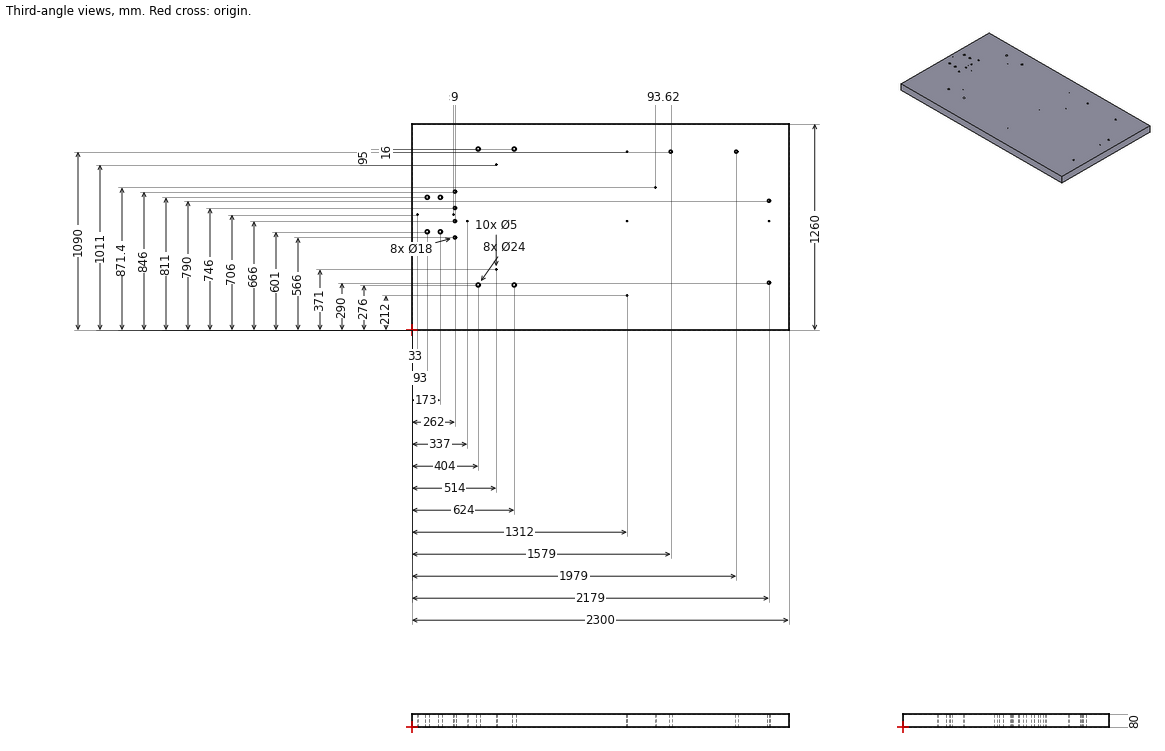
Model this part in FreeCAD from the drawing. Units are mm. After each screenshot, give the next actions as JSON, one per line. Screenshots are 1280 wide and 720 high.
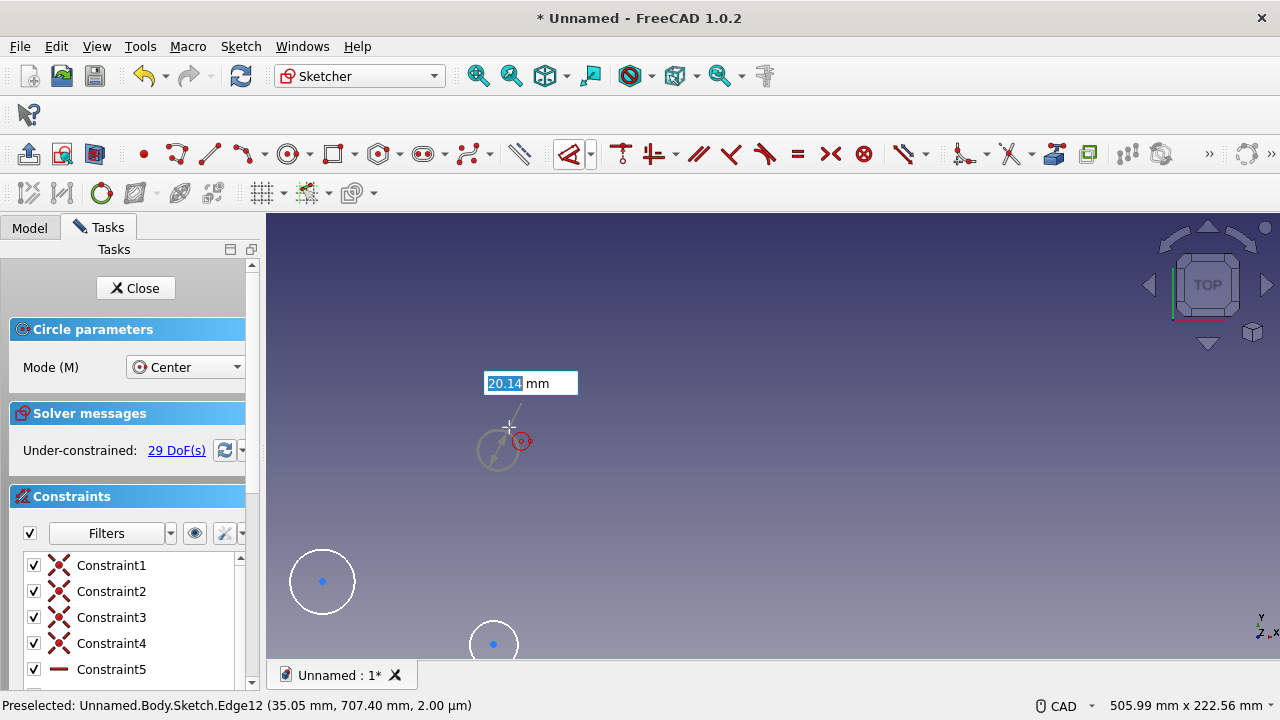
{"action": "left_click", "coordinate": [510, 425]}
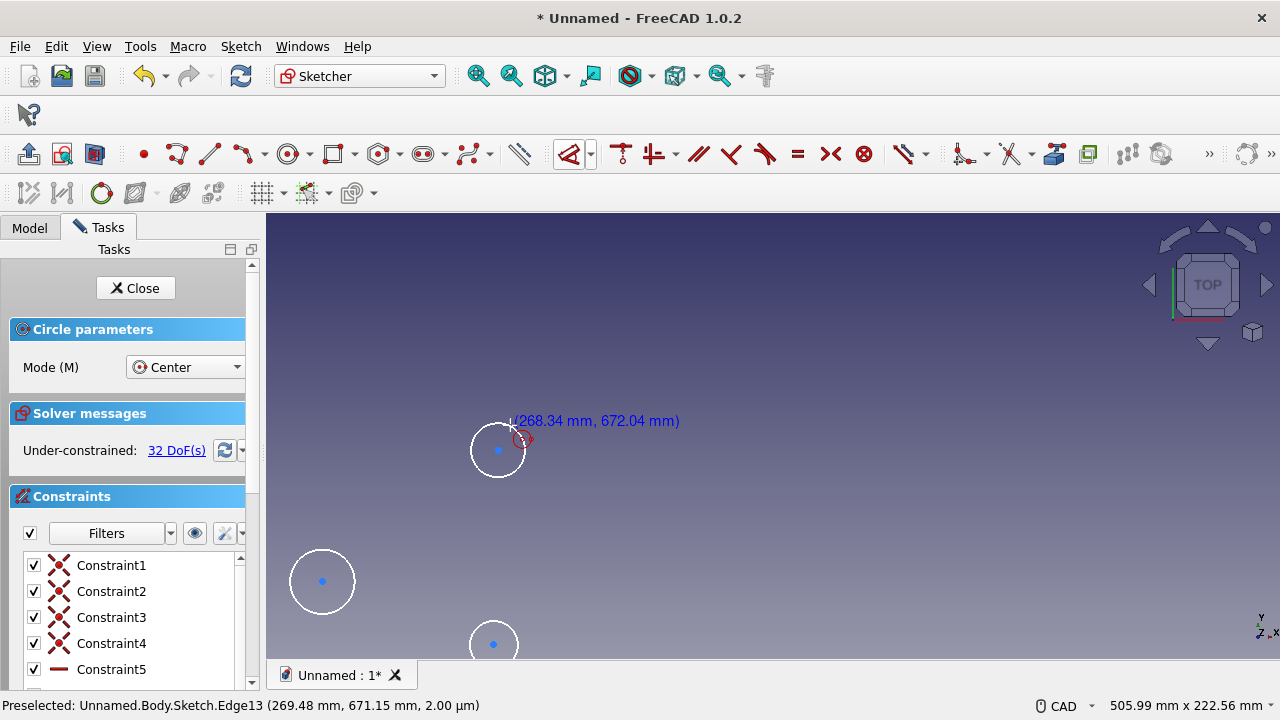
{"action": "scroll", "coordinate": [479, 358], "scroll_direction": "up", "scroll_amount": 8}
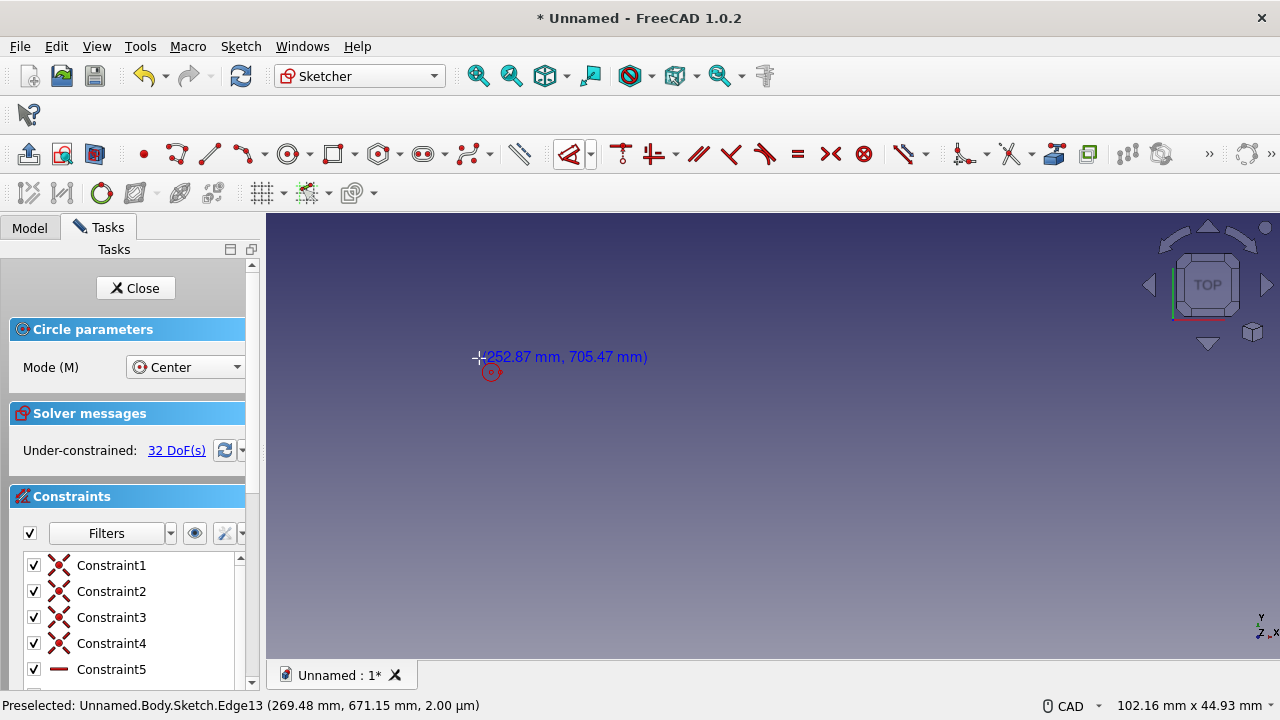
{"action": "scroll", "coordinate": [704, 436], "scroll_direction": "down", "scroll_amount": 15}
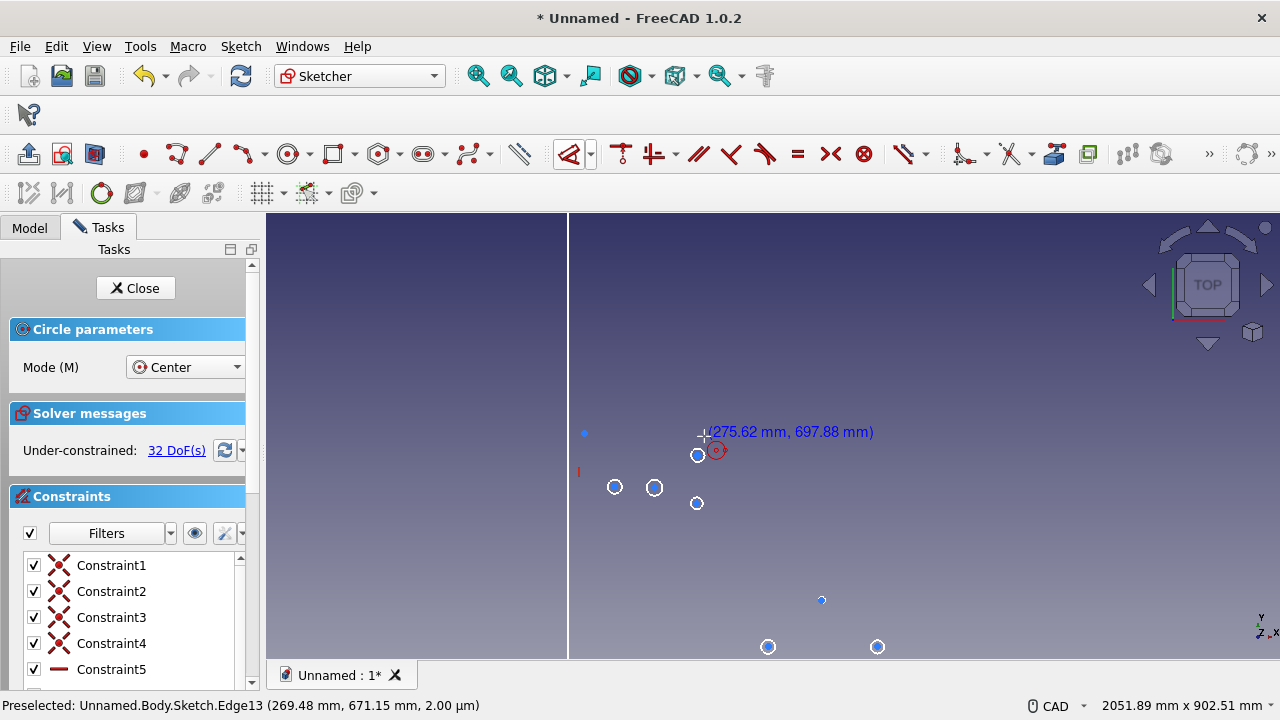
{"action": "scroll", "coordinate": [352, 408], "scroll_direction": "down", "scroll_amount": 4}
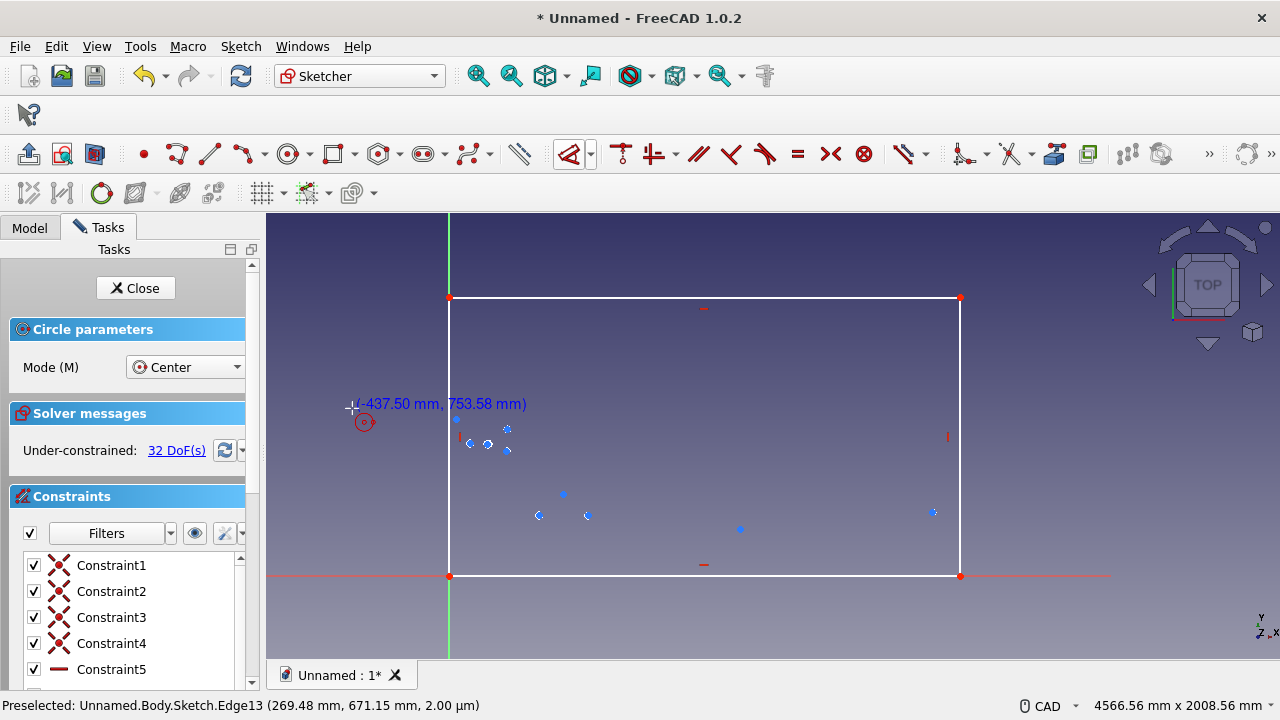
{"action": "scroll", "coordinate": [505, 419], "scroll_direction": "up", "scroll_amount": 5}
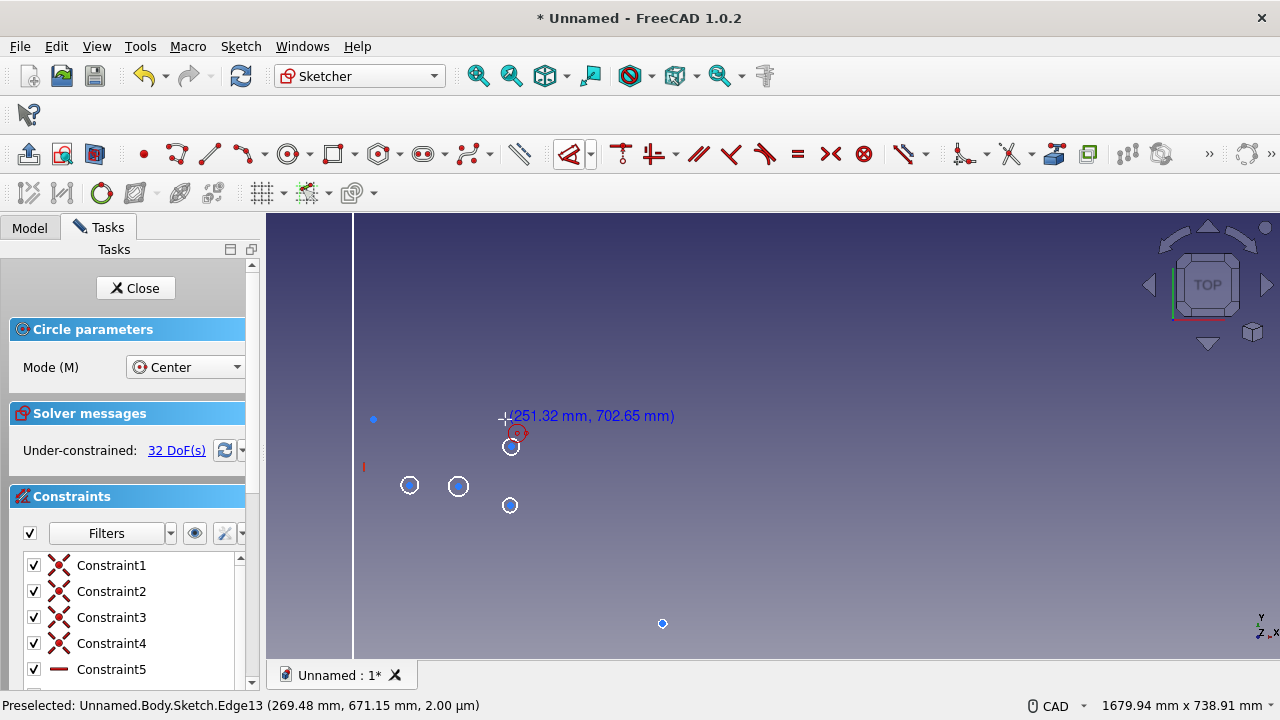
{"action": "left_click", "coordinate": [506, 419]}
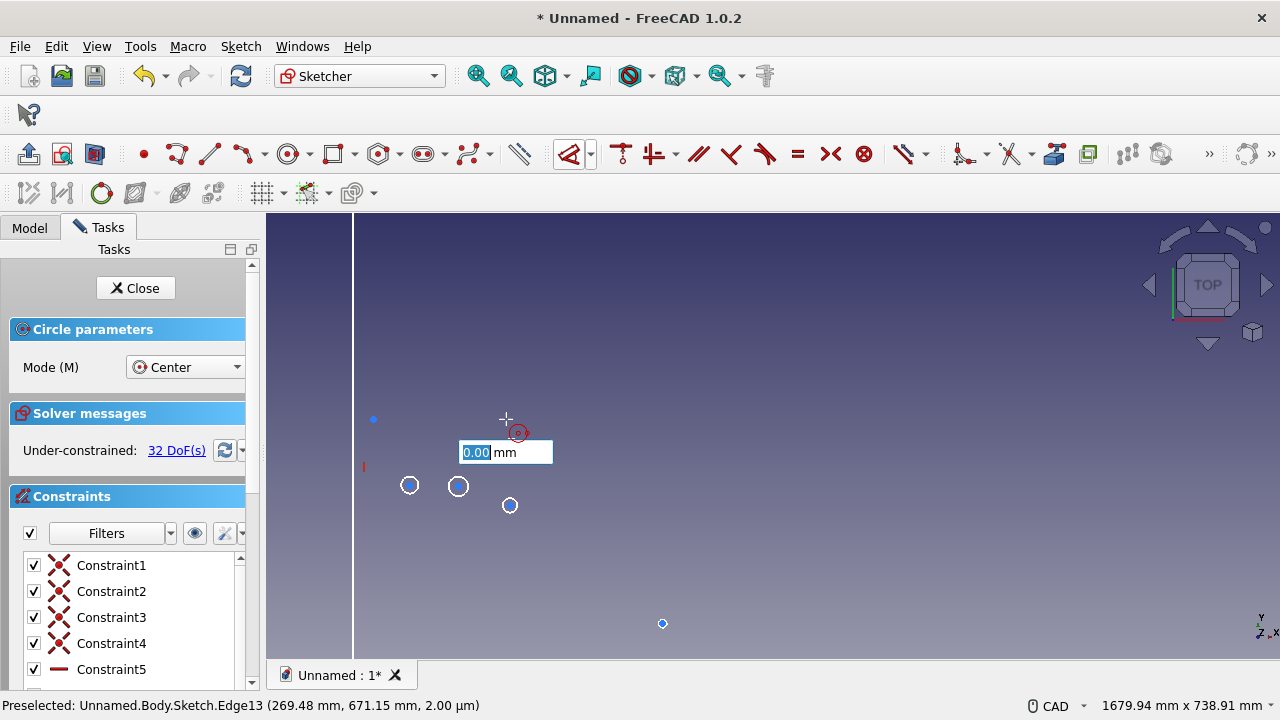
{"action": "scroll", "coordinate": [507, 418], "scroll_direction": "up", "scroll_amount": 12}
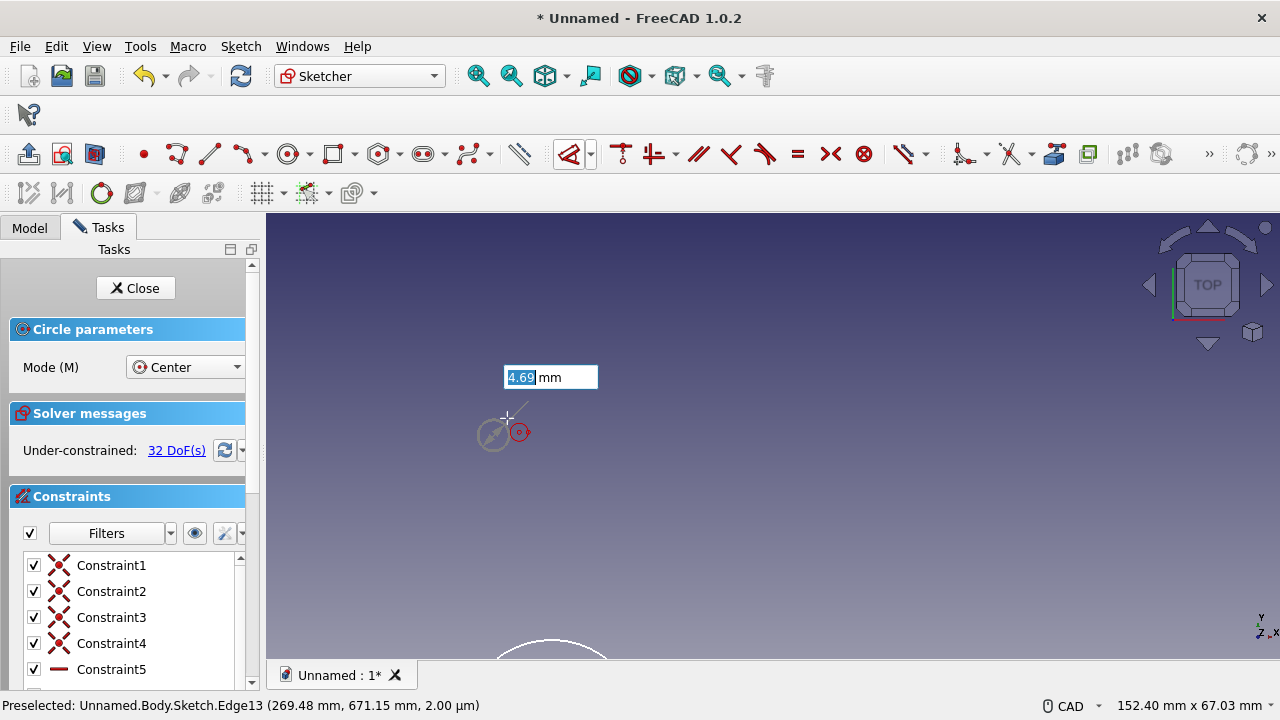
{"action": "left_click", "coordinate": [501, 412]}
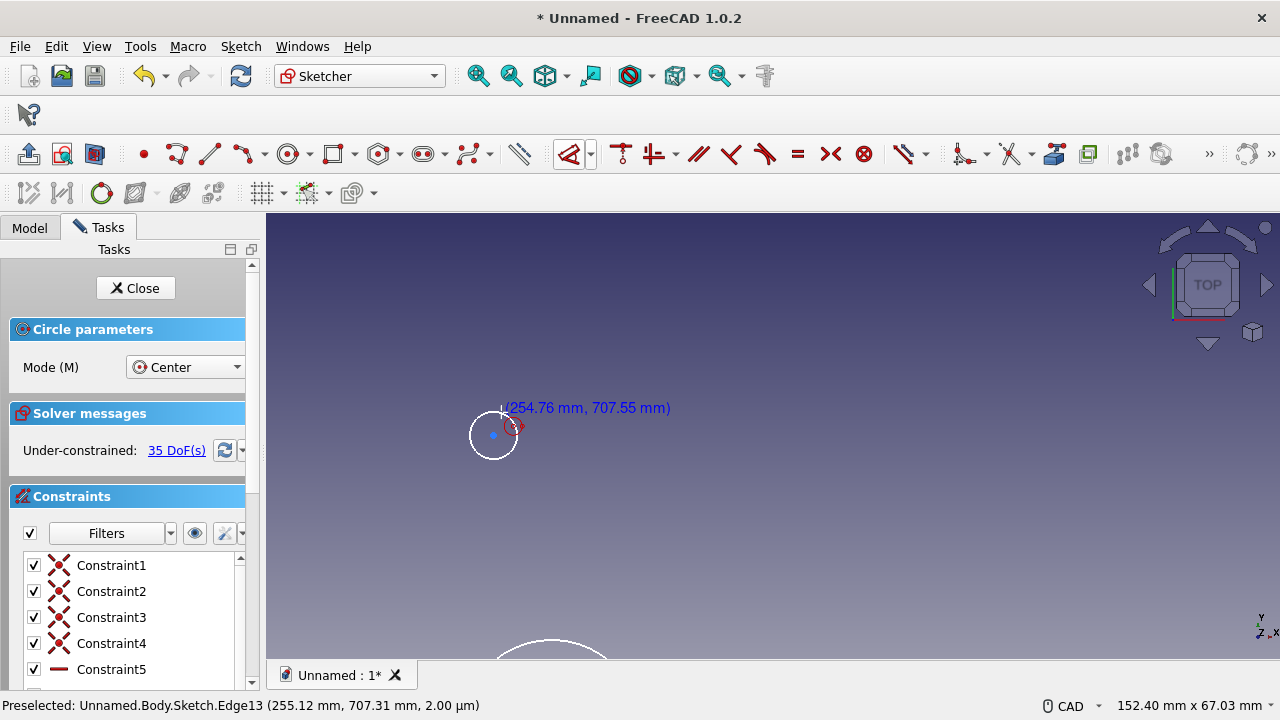
{"action": "scroll", "coordinate": [506, 419], "scroll_direction": "down", "scroll_amount": 17}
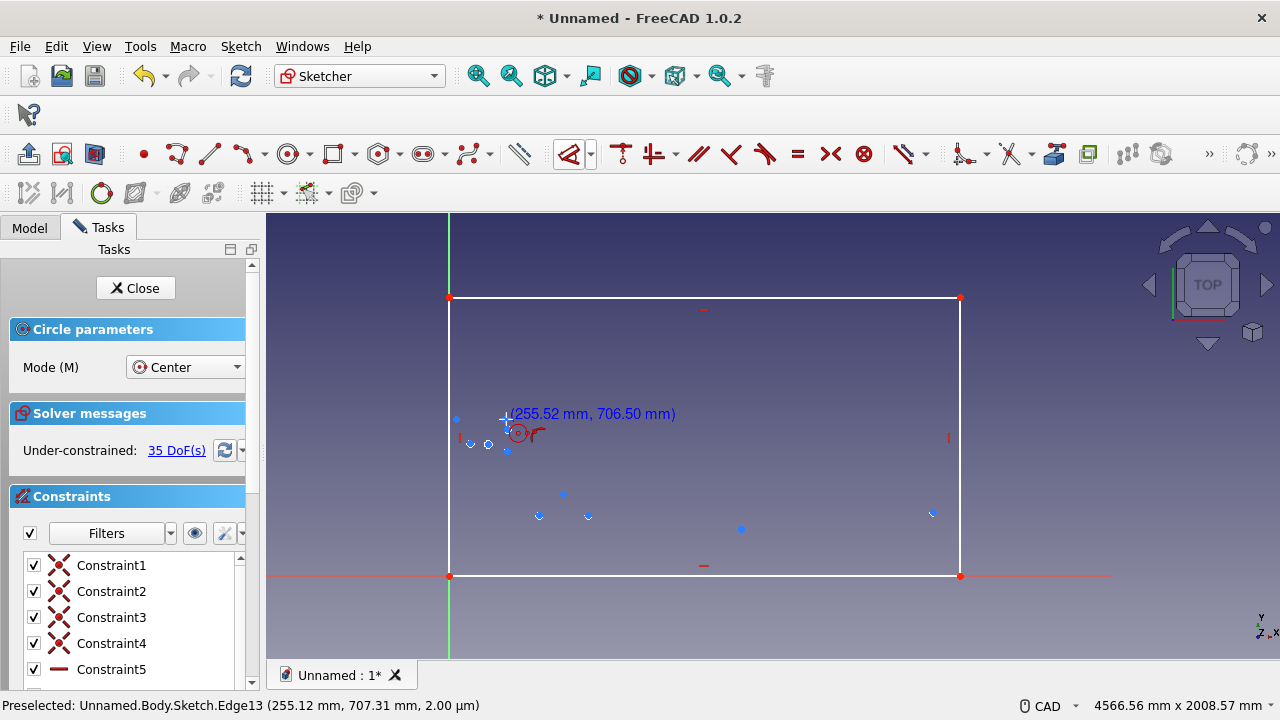
{"action": "scroll", "coordinate": [508, 411], "scroll_direction": "up", "scroll_amount": 13}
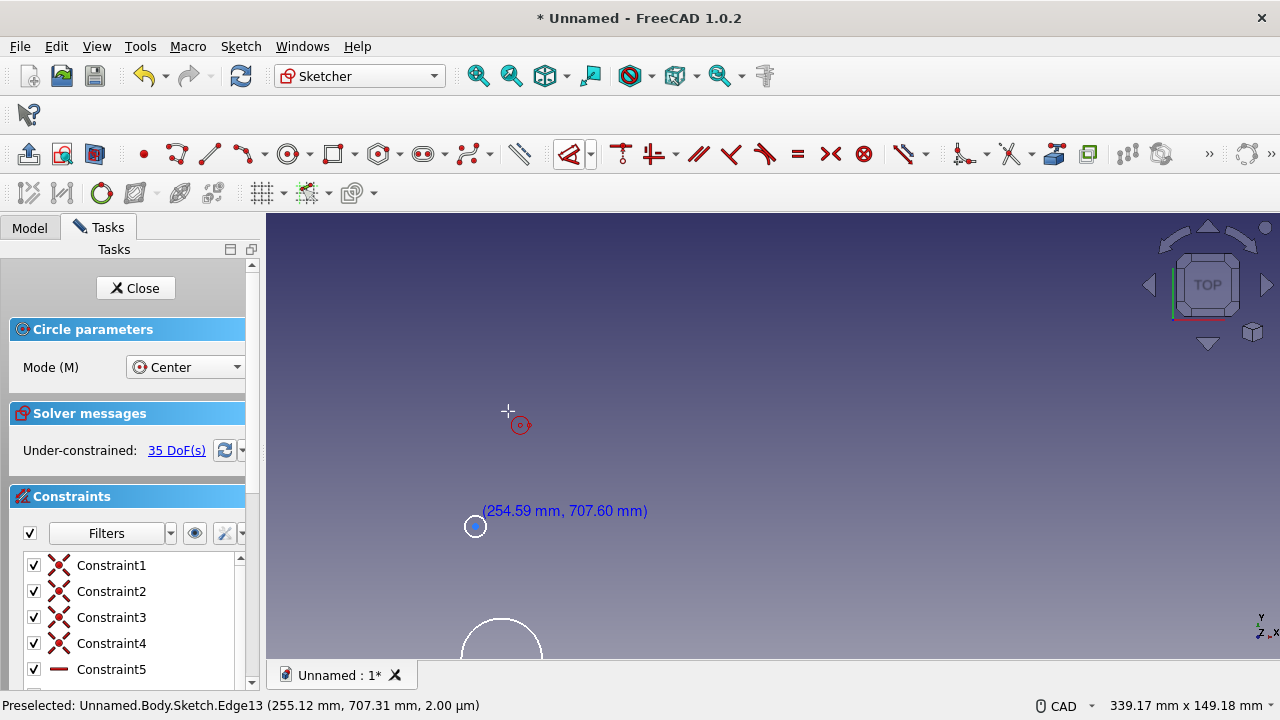
{"action": "scroll", "coordinate": [508, 411], "scroll_direction": "down", "scroll_amount": 13}